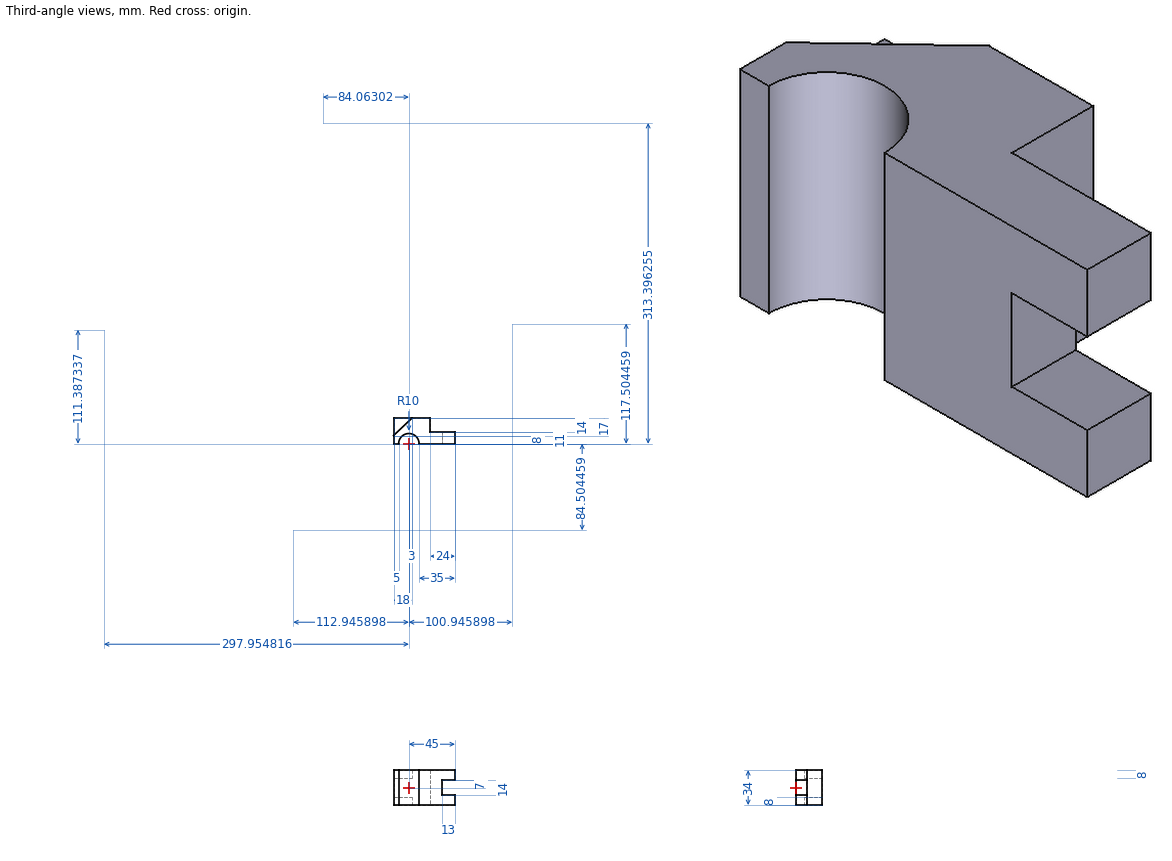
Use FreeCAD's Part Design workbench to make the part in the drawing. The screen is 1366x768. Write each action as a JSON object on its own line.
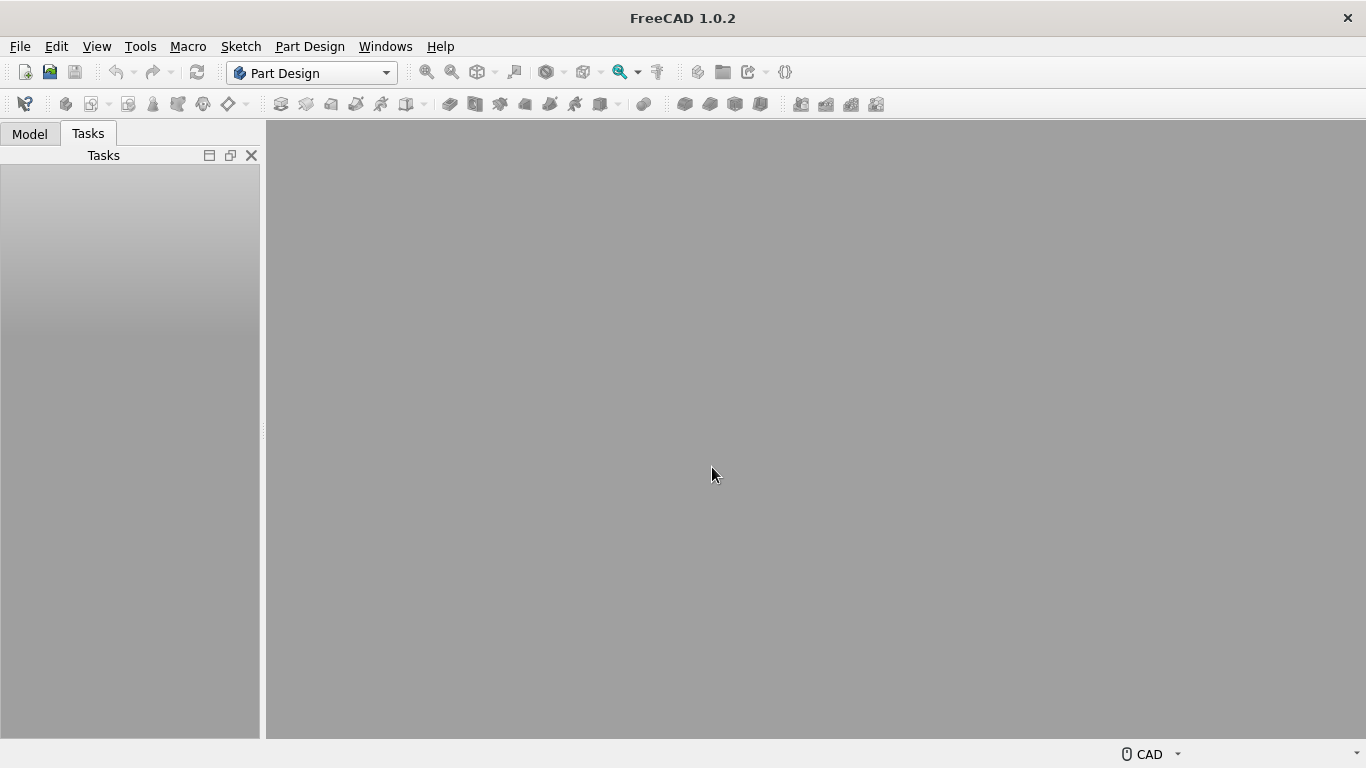
{"action": "left_click", "coordinate": [25, 72]}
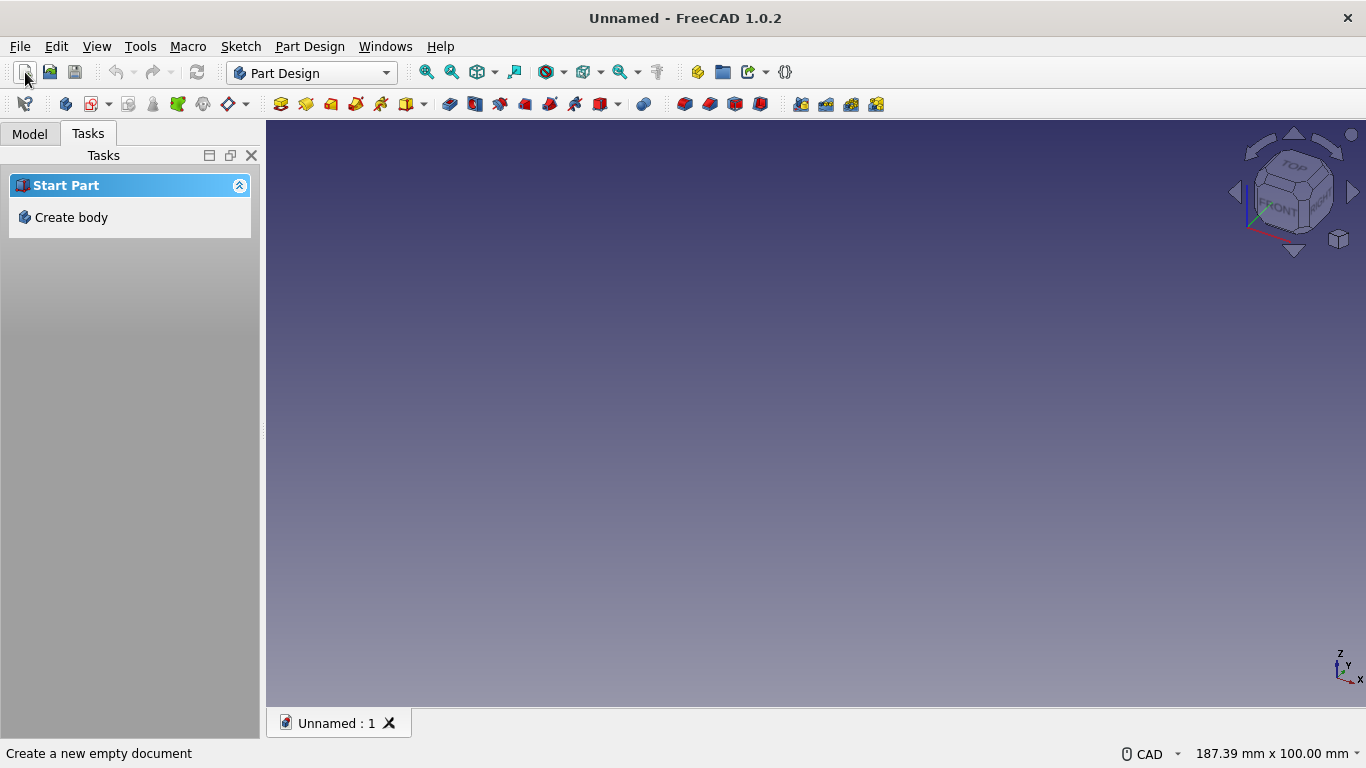
{"action": "left_click", "coordinate": [90, 104]}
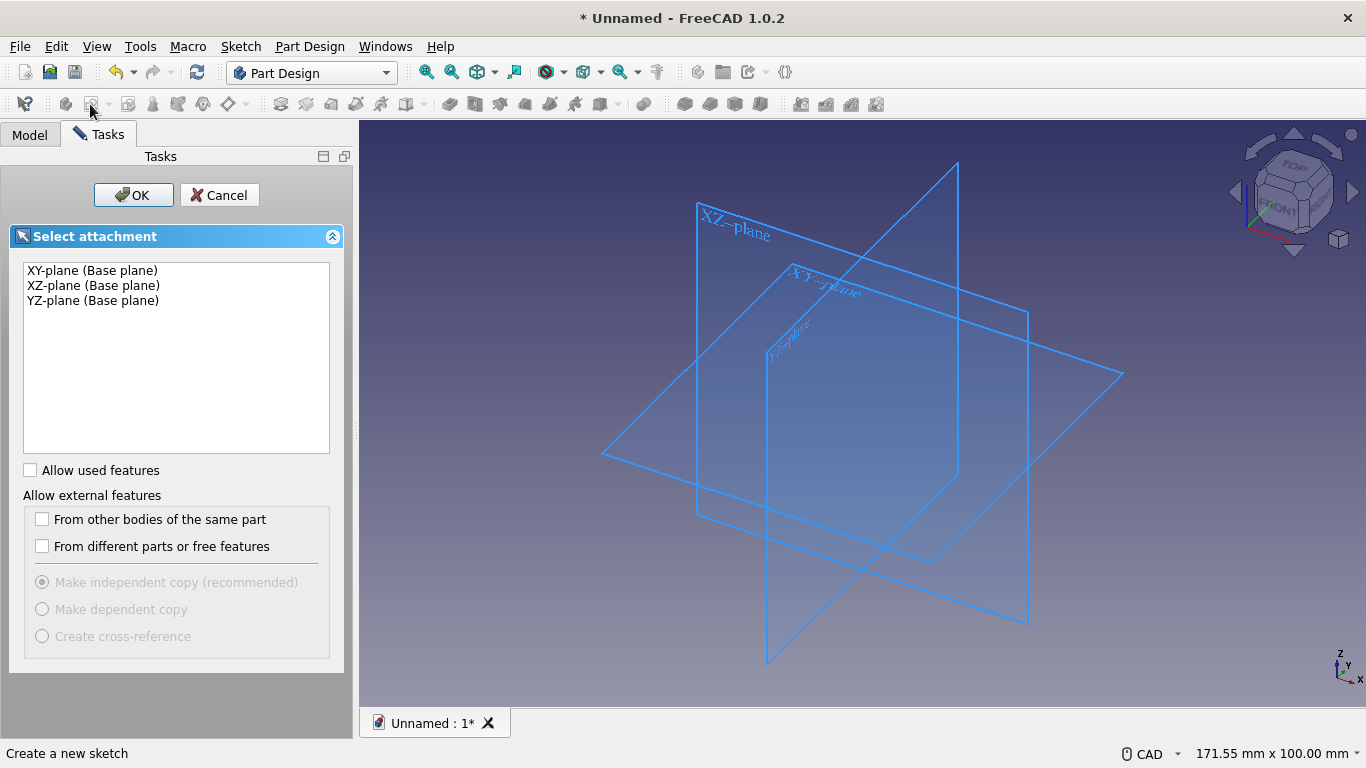
{"action": "left_click", "coordinate": [84, 270]}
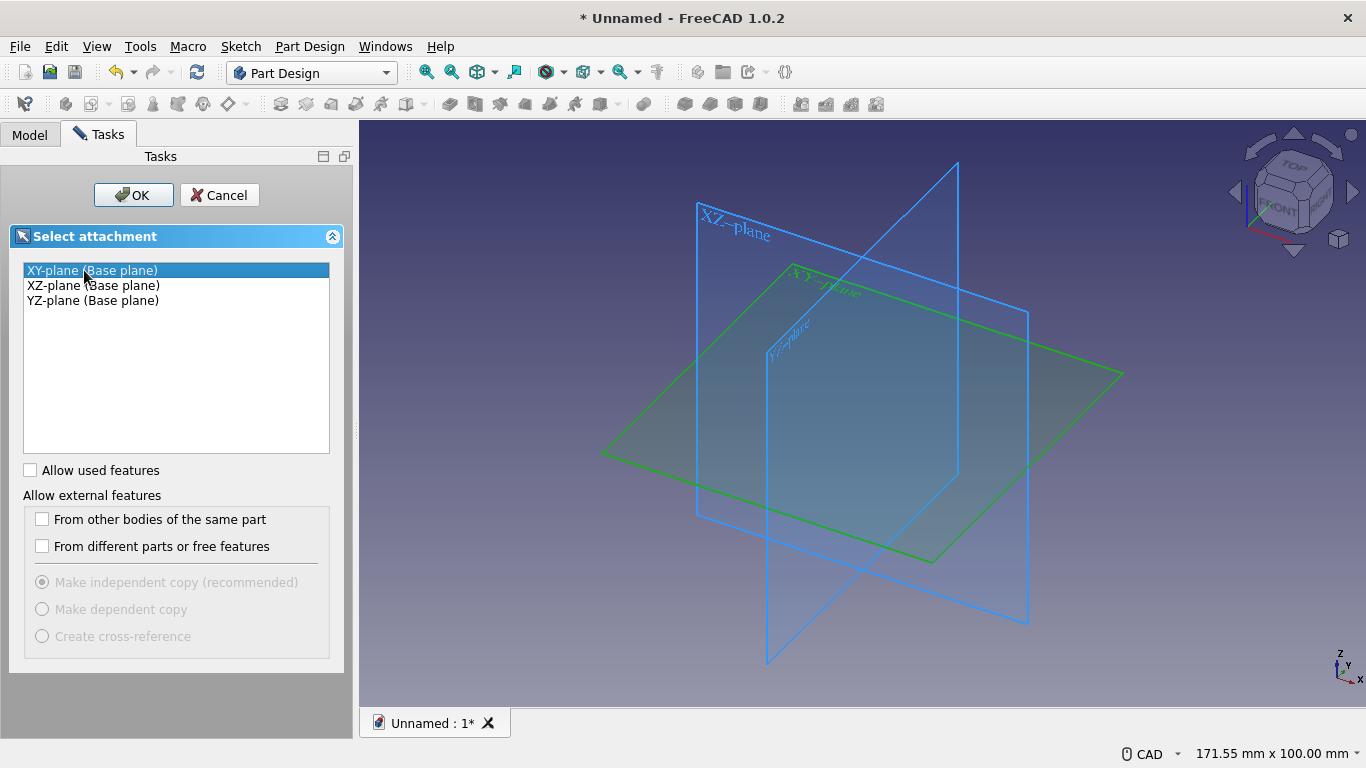
{"action": "left_click", "coordinate": [134, 195]}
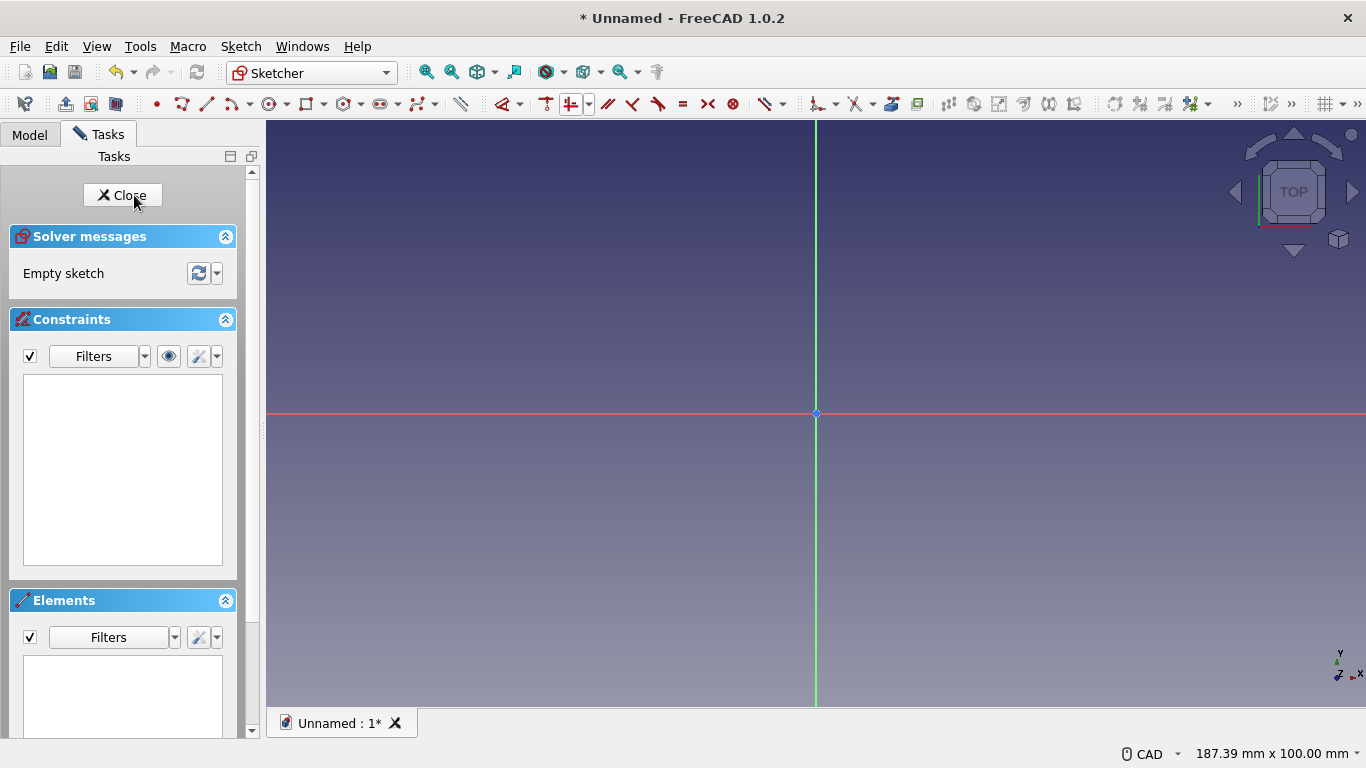
{"action": "scroll", "coordinate": [1094, 251], "scroll_direction": "up", "scroll_amount": 3}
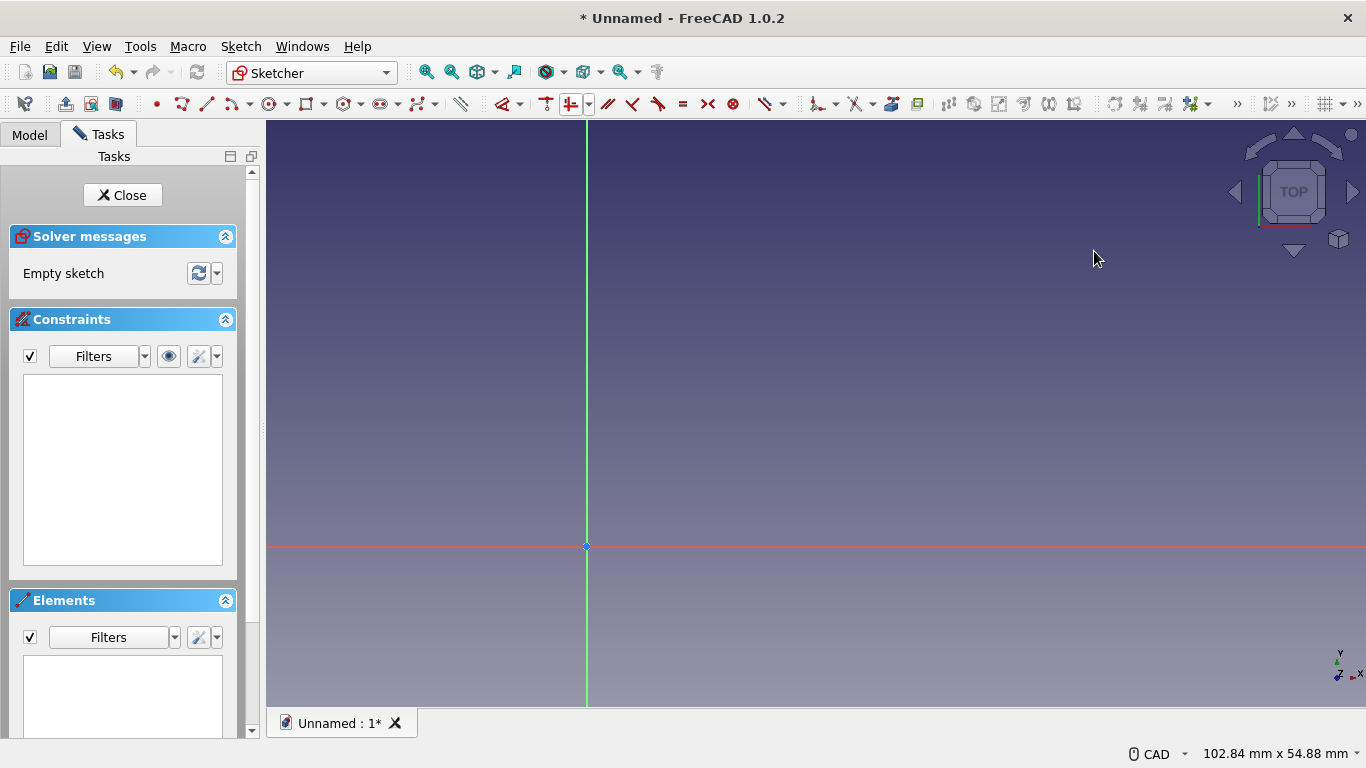
{"action": "left_click", "coordinate": [182, 104]}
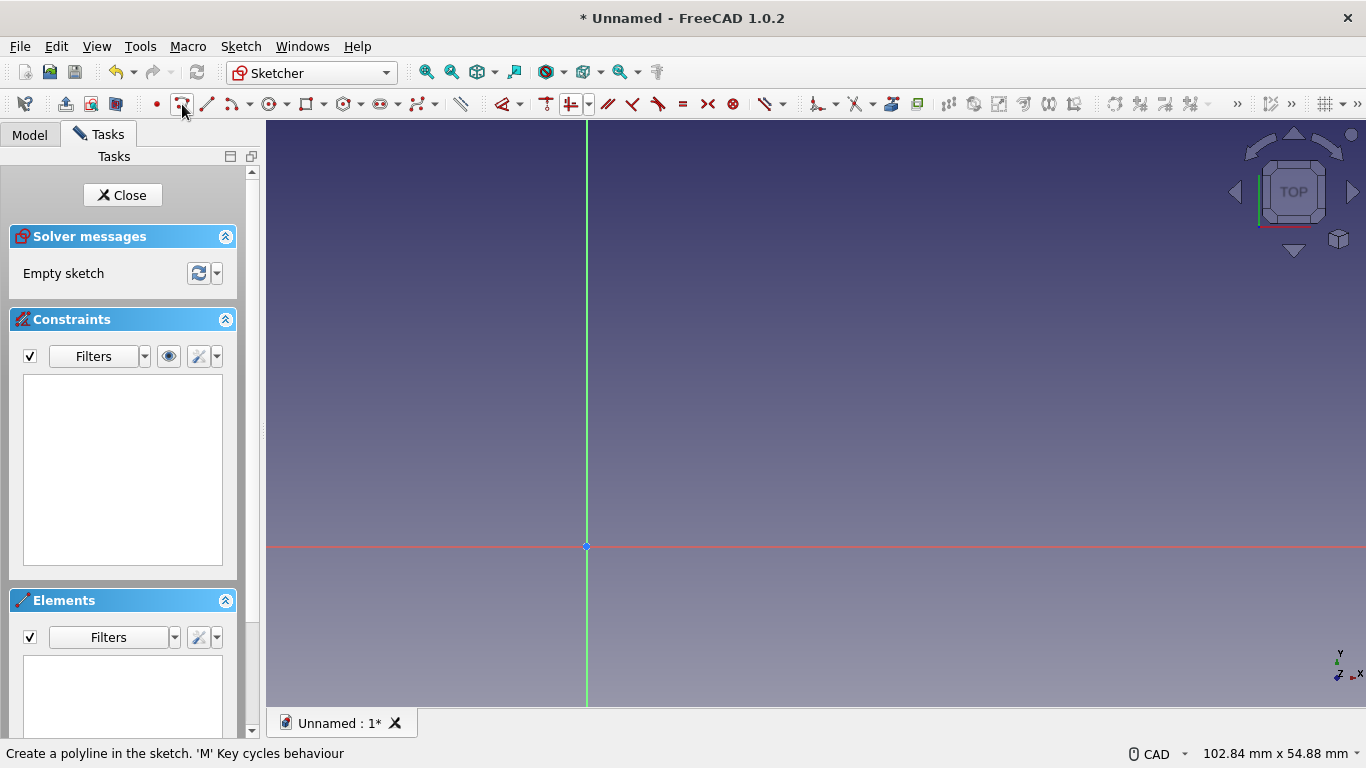
{"action": "left_click", "coordinate": [694, 547]}
{"action": "left_click", "coordinate": [1068, 538]}
{"action": "left_click", "coordinate": [1068, 429]}
{"action": "left_click", "coordinate": [811, 429]}
{"action": "left_click", "coordinate": [811, 280]}
{"action": "left_click", "coordinate": [426, 280]}
{"action": "left_click", "coordinate": [426, 547]}
{"action": "left_click", "coordinate": [480, 538]}
{"action": "right_click", "coordinate": [480, 538]}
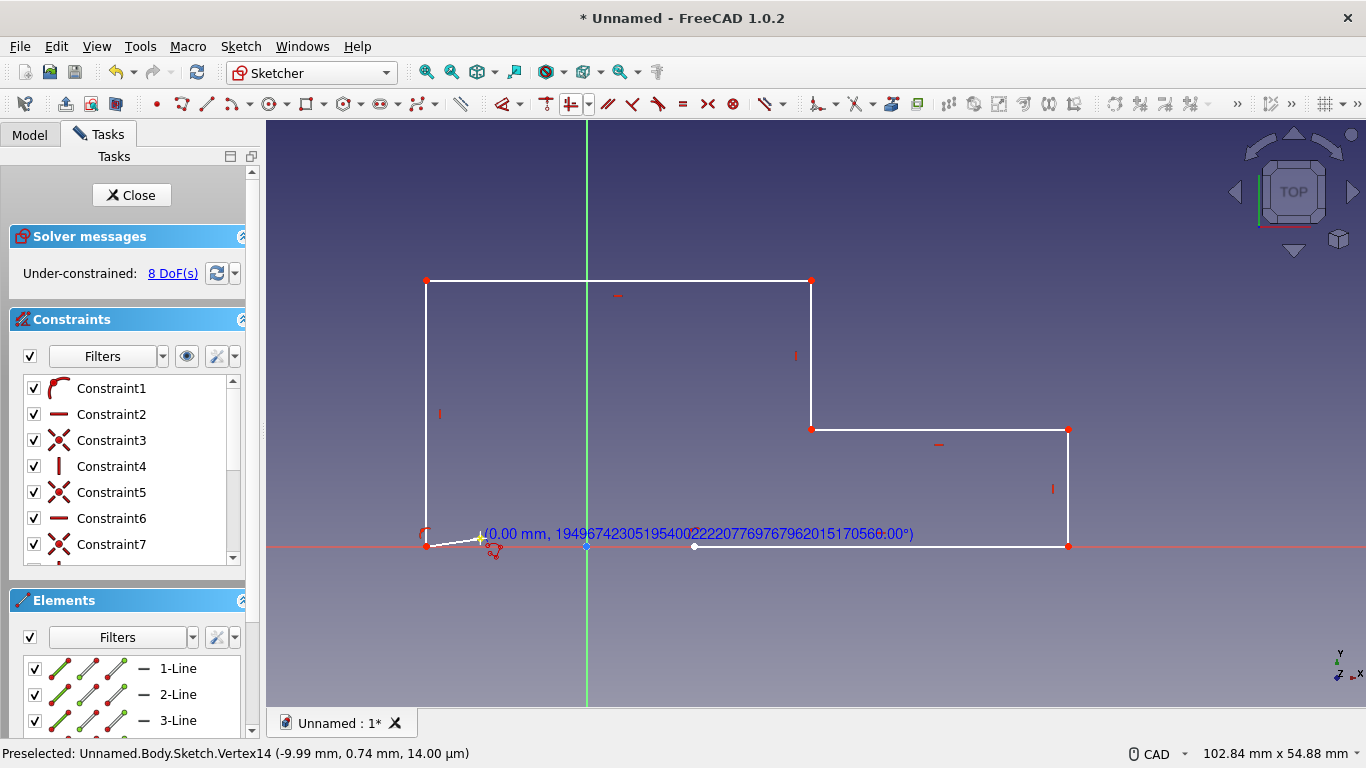
{"action": "left_click", "coordinate": [250, 104]}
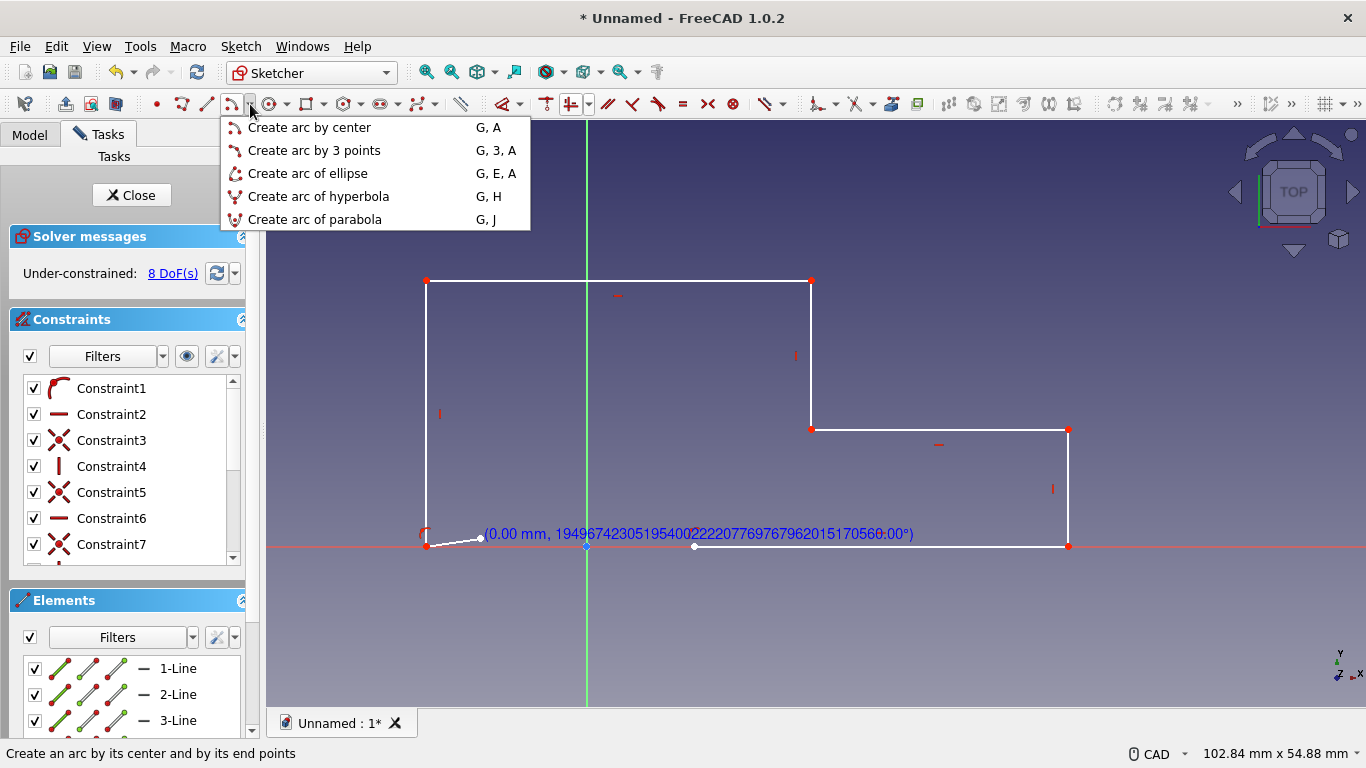
{"action": "left_click", "coordinate": [376, 150]}